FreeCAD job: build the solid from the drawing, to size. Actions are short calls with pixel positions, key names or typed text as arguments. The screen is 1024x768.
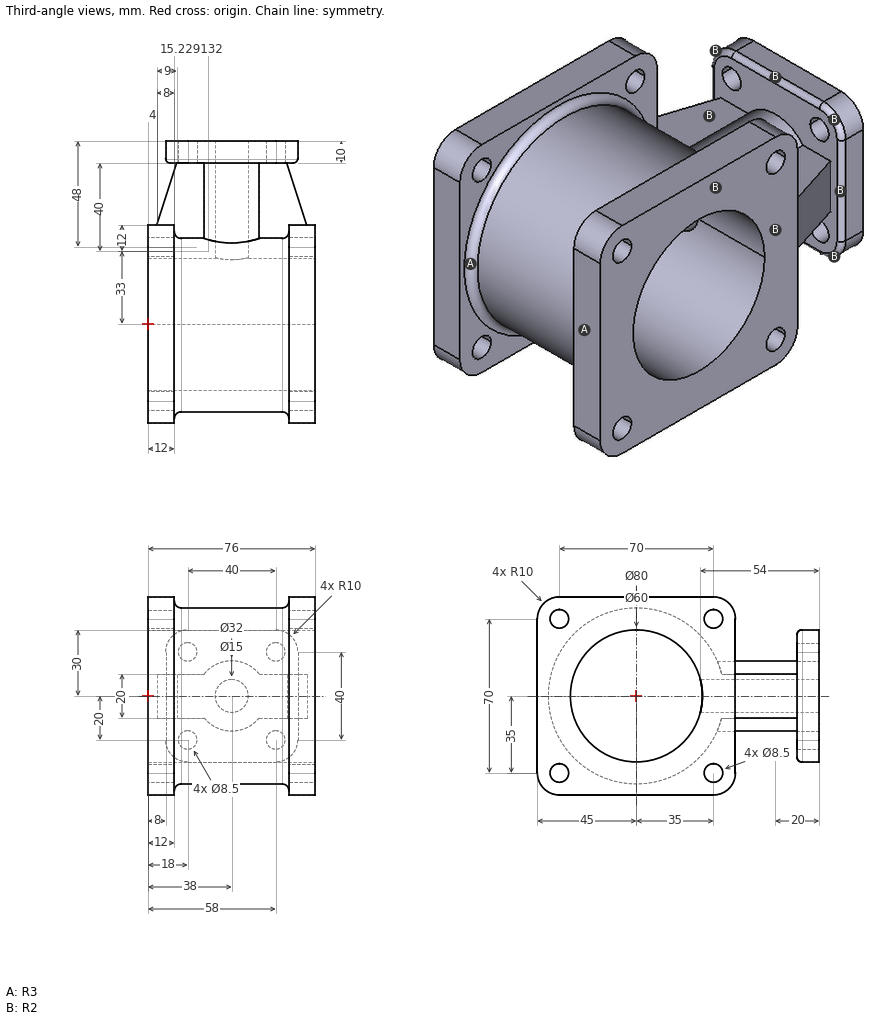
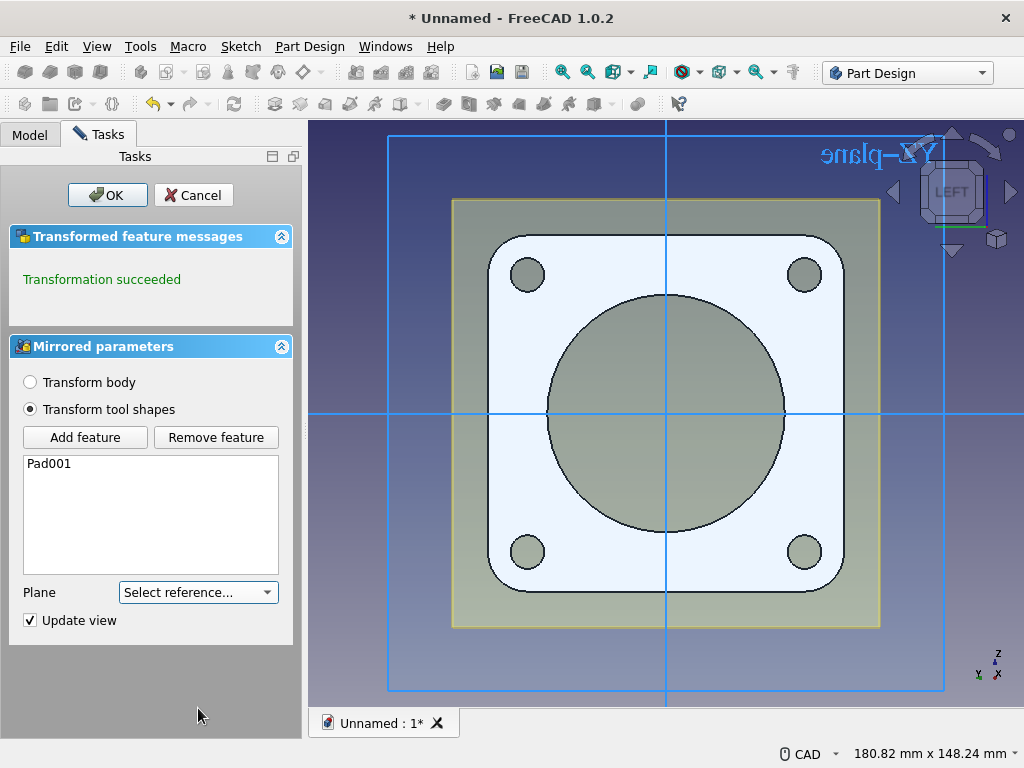
click(30, 134)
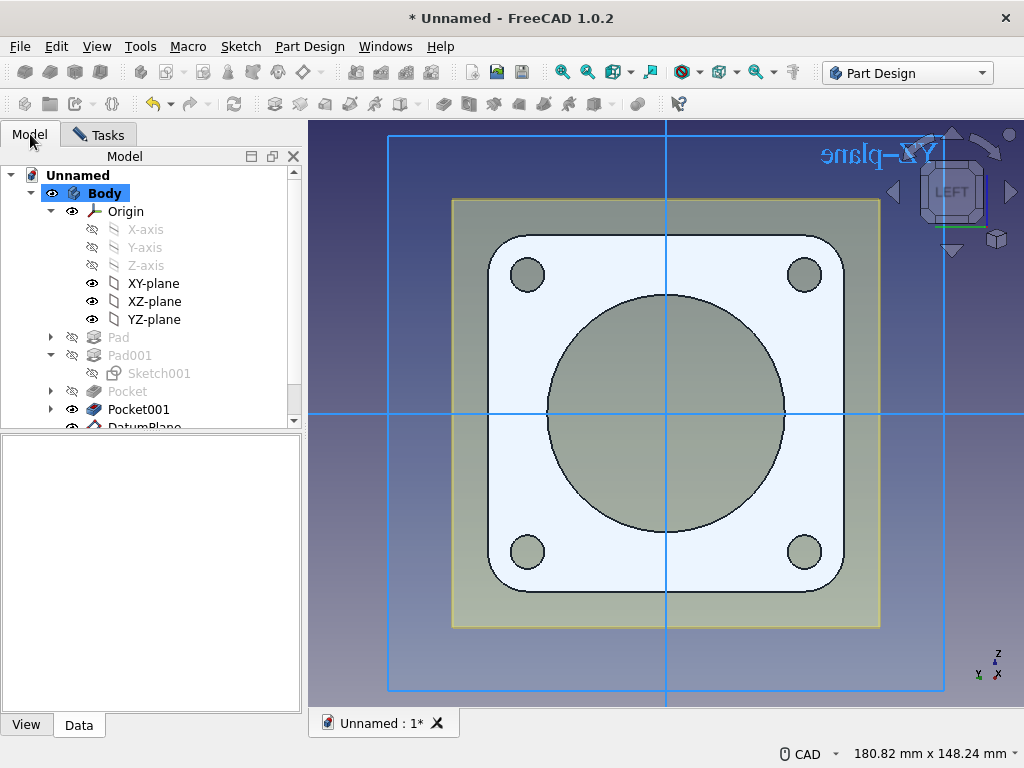
click(117, 427)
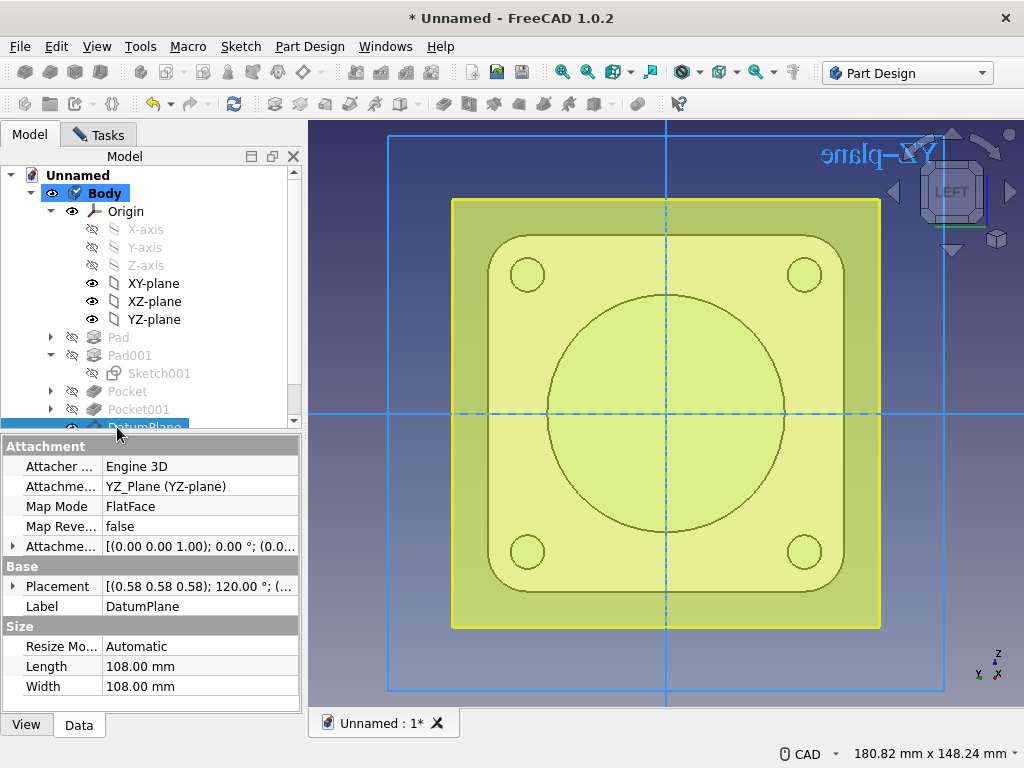
click(98, 134)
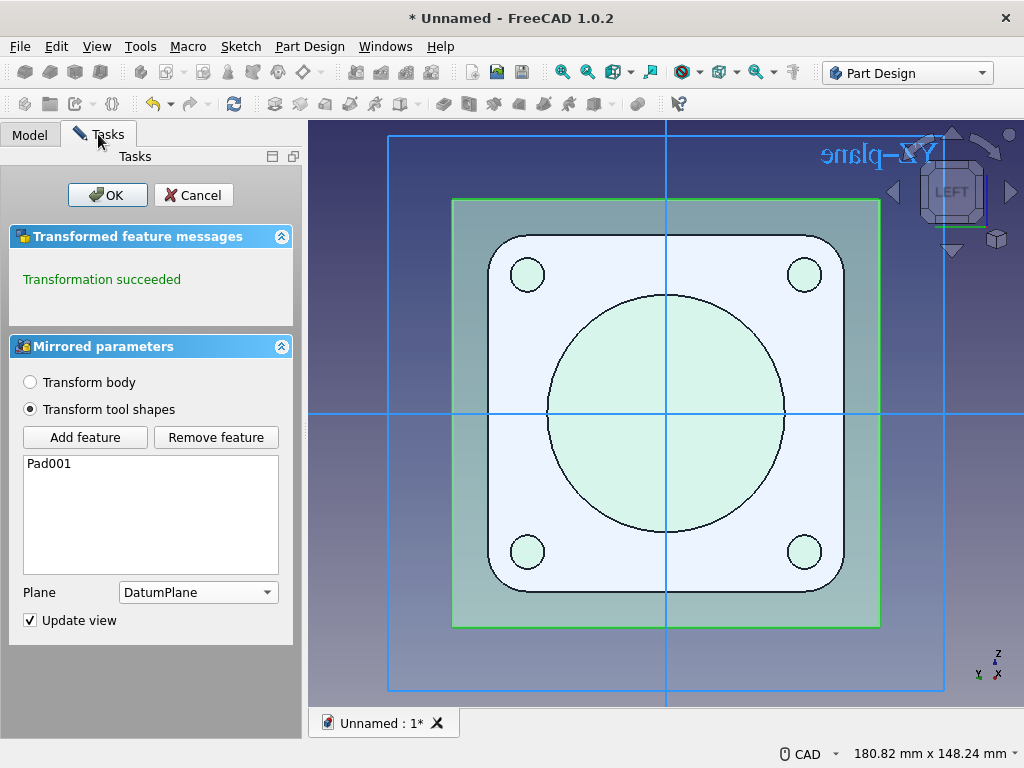
click(108, 195)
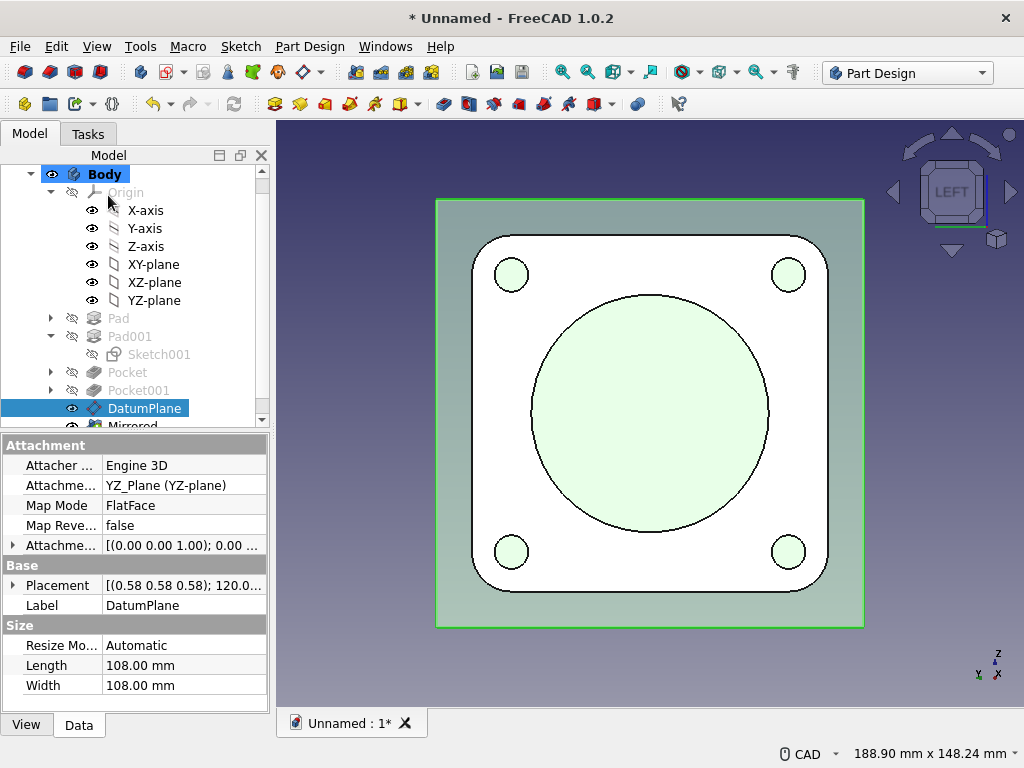
click(117, 408)
key(space)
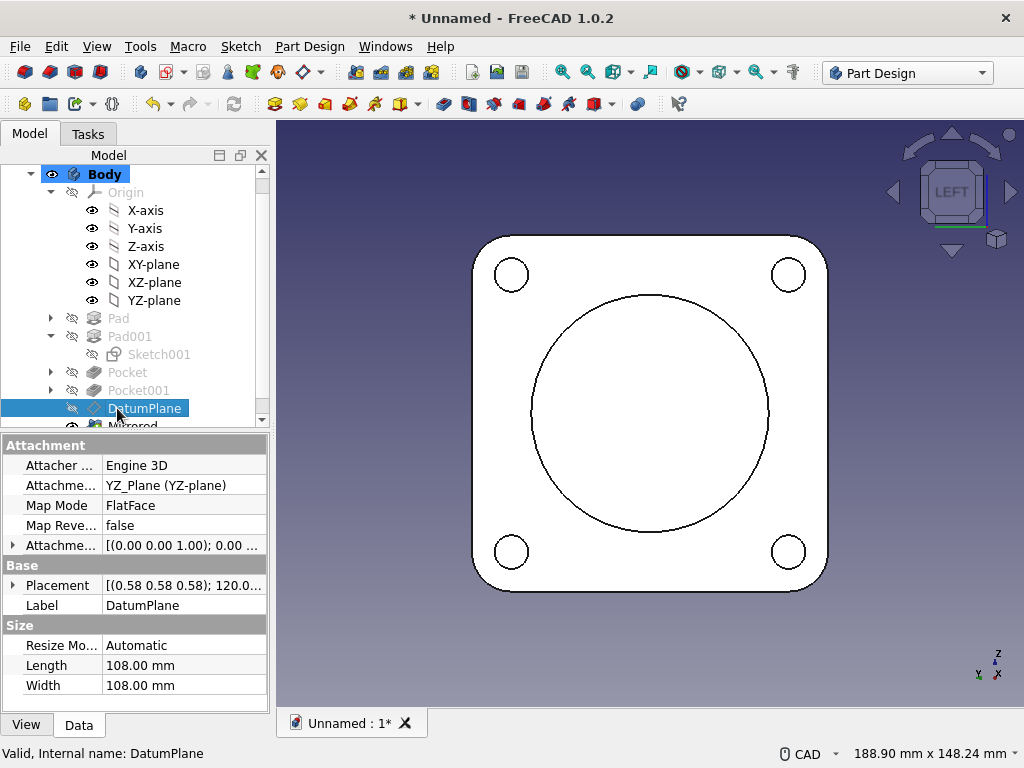
click(137, 300)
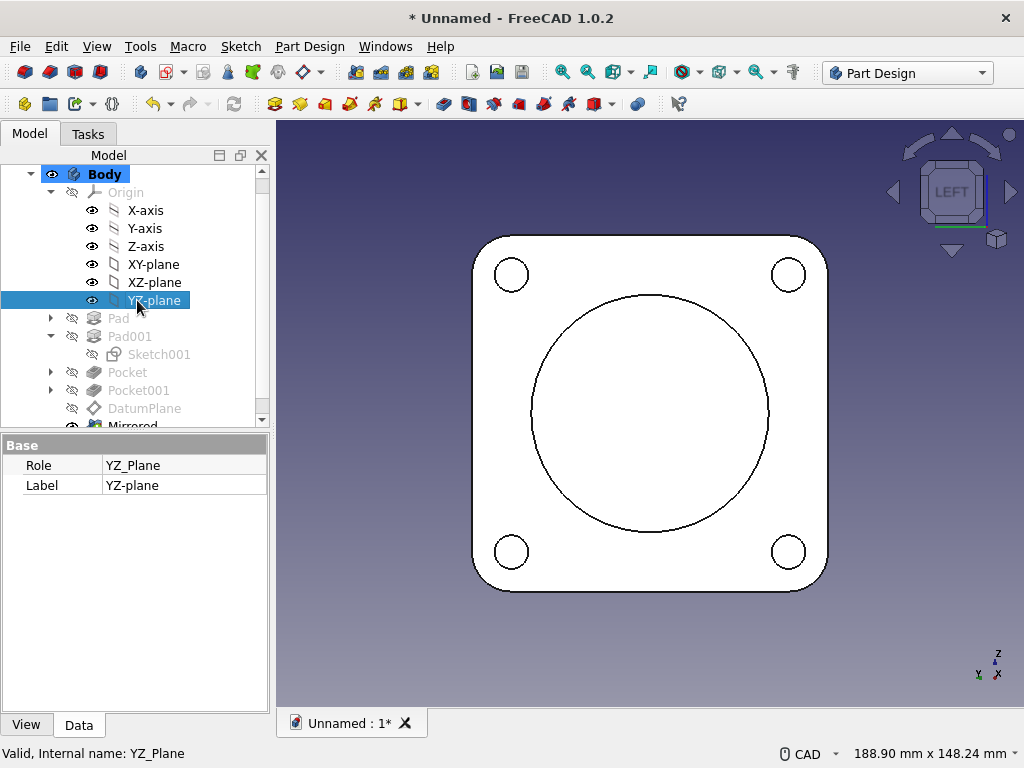
click(302, 72)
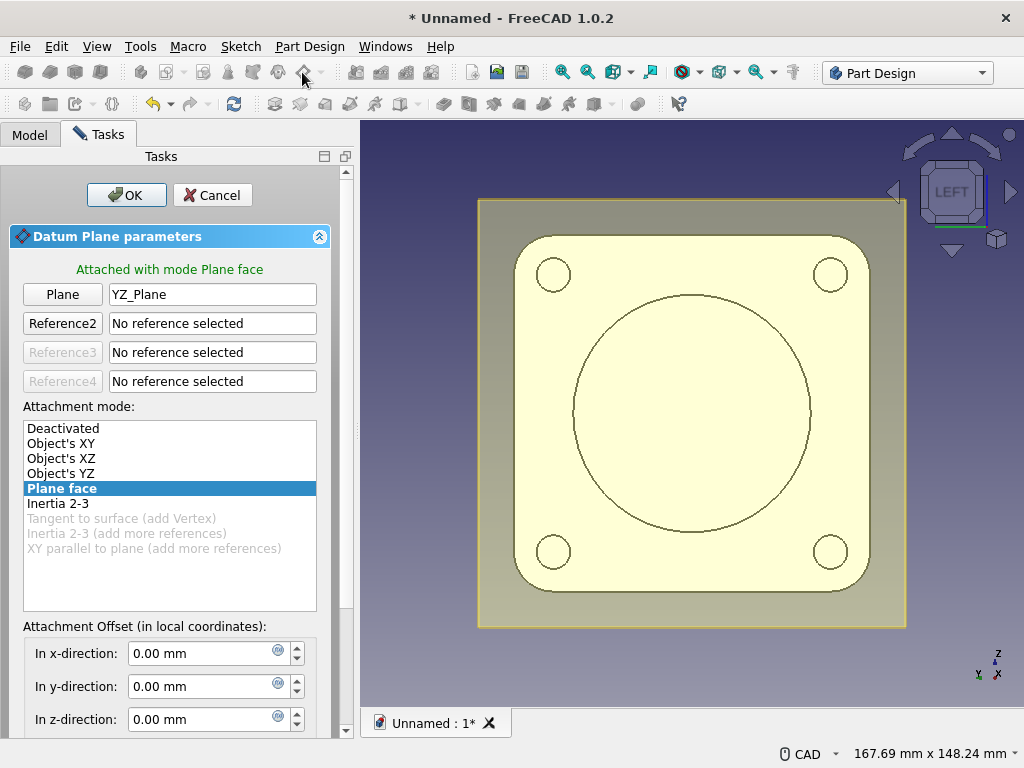
triple_click(210, 720)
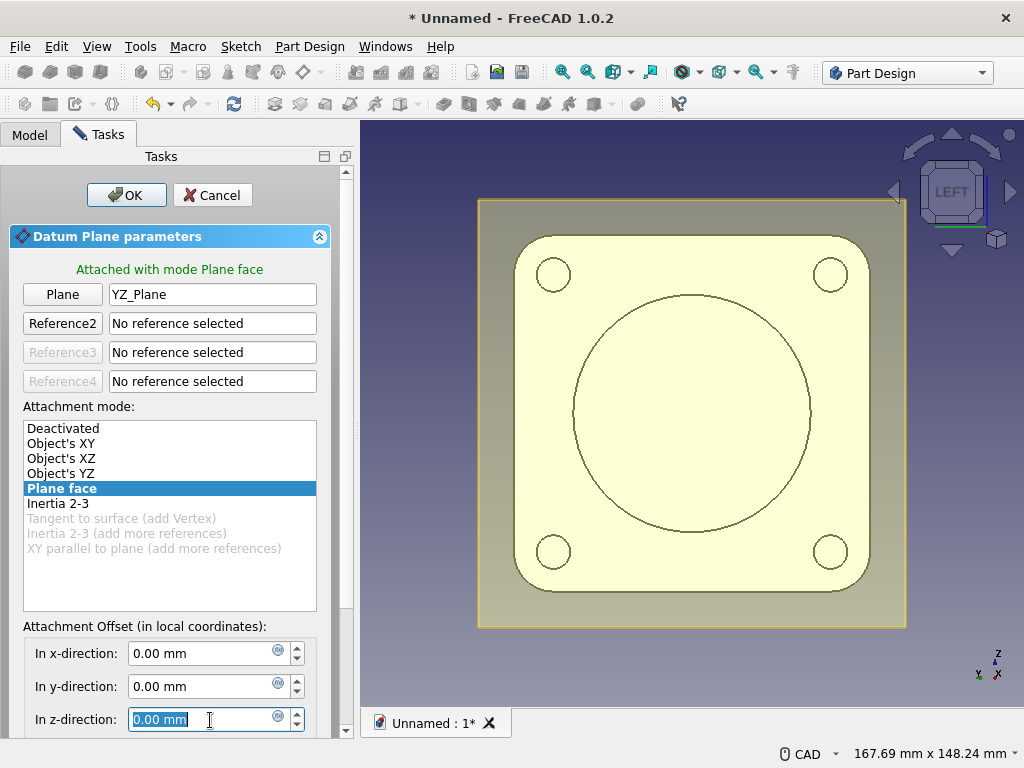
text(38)
key(Tab)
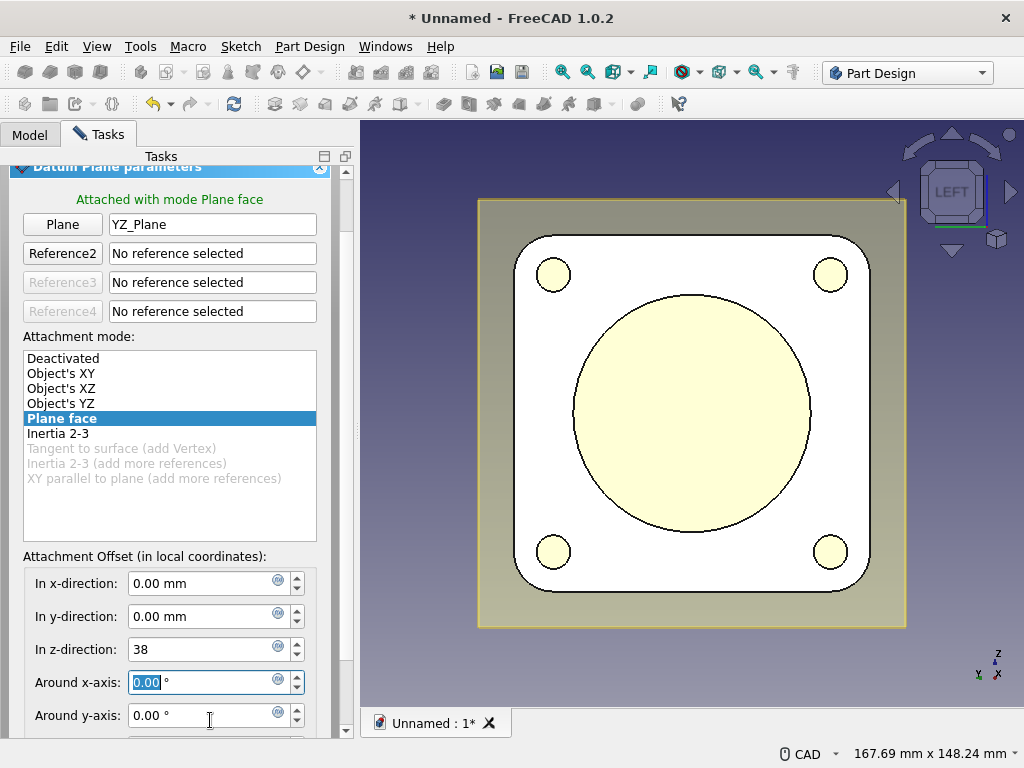
scroll(346, 452, up, 2)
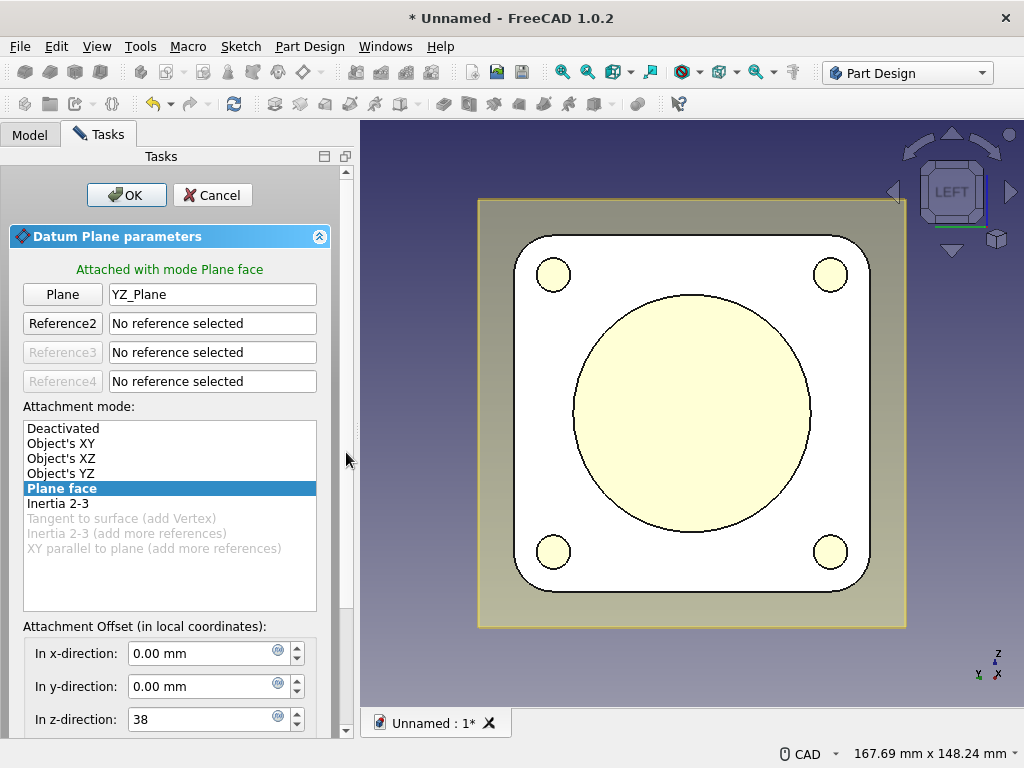
click(127, 195)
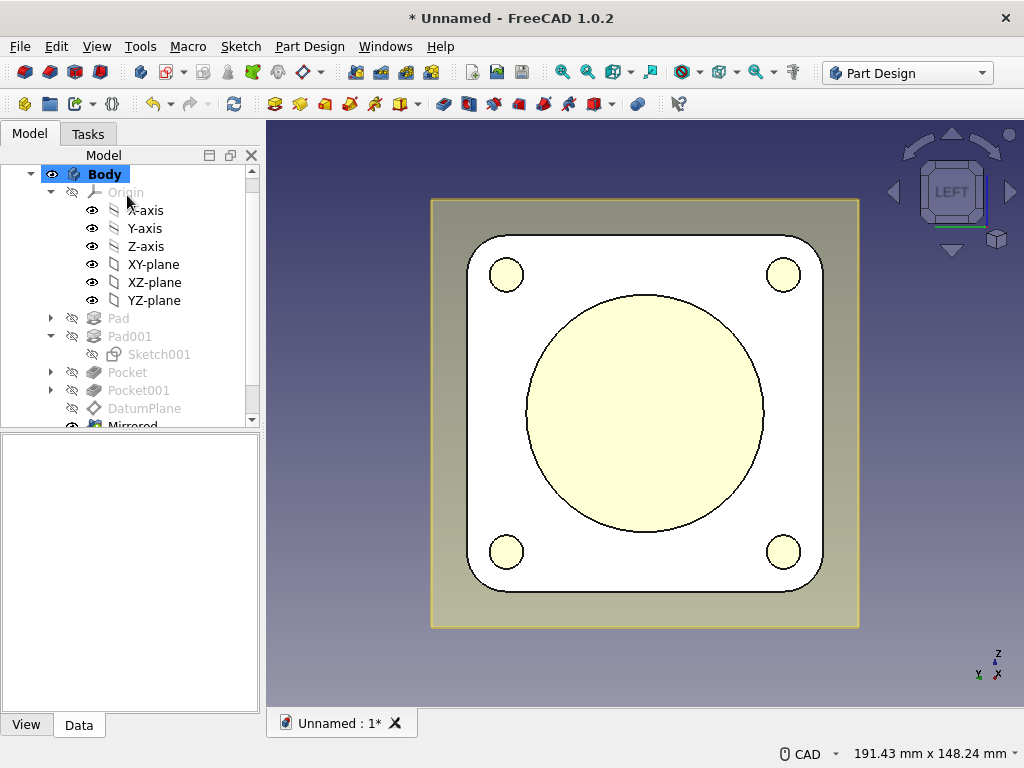
click(117, 372)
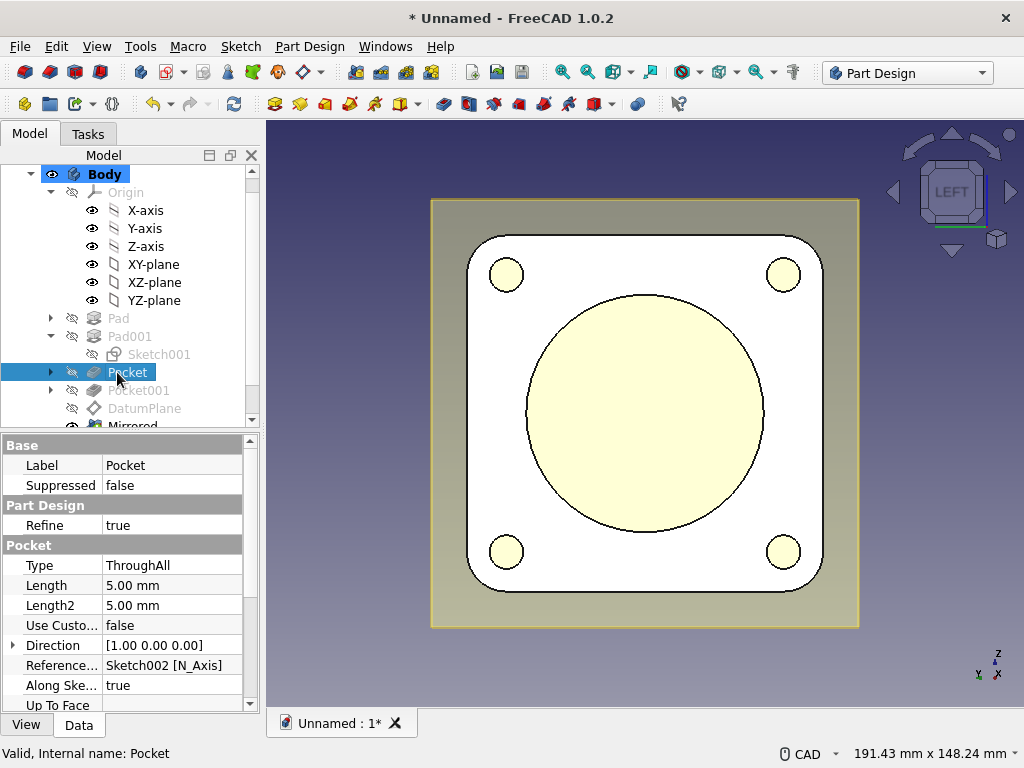
click(117, 390, ctrl)